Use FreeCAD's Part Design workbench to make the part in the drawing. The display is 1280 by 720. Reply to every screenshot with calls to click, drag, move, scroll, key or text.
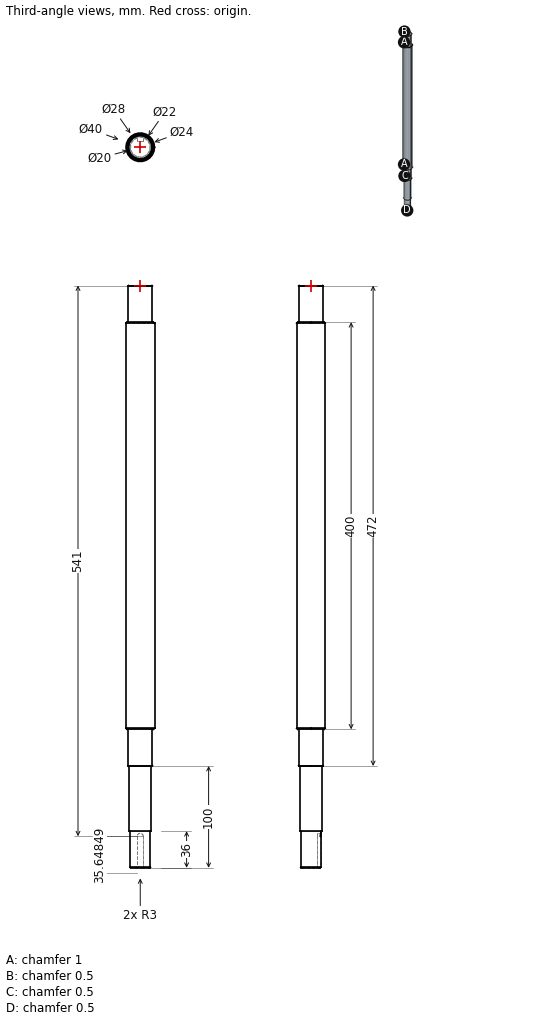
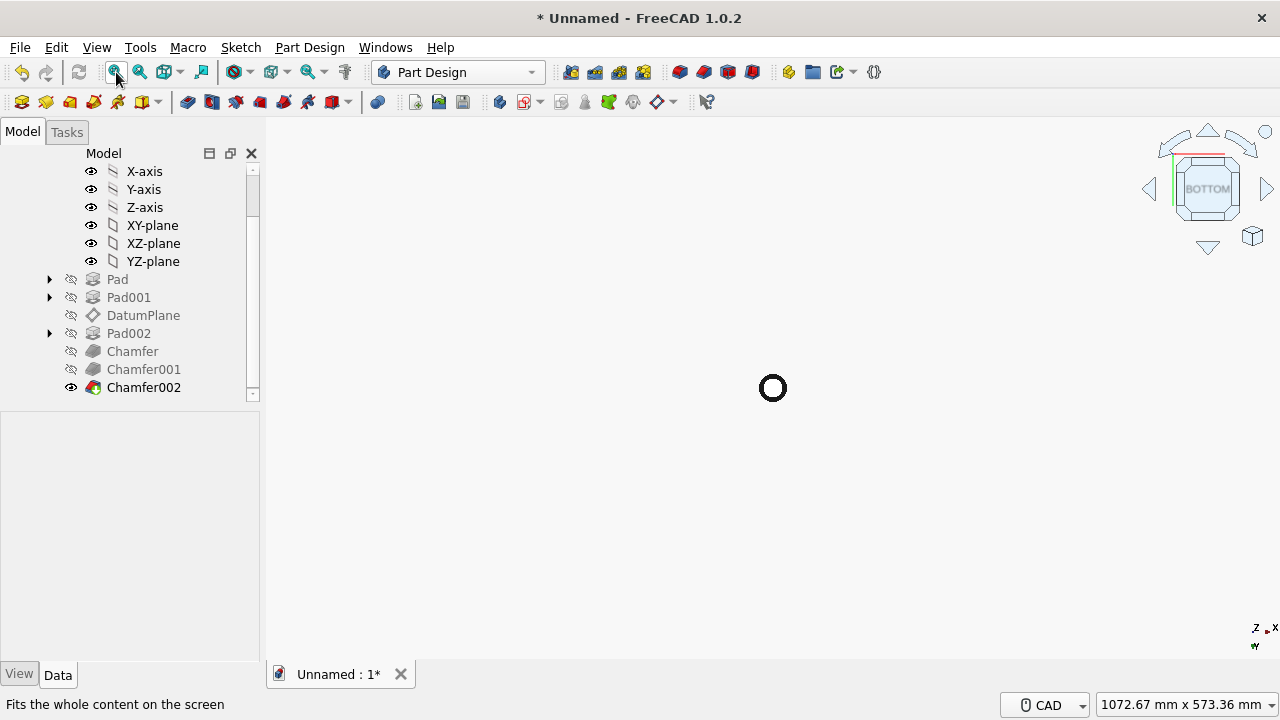
click(773, 387)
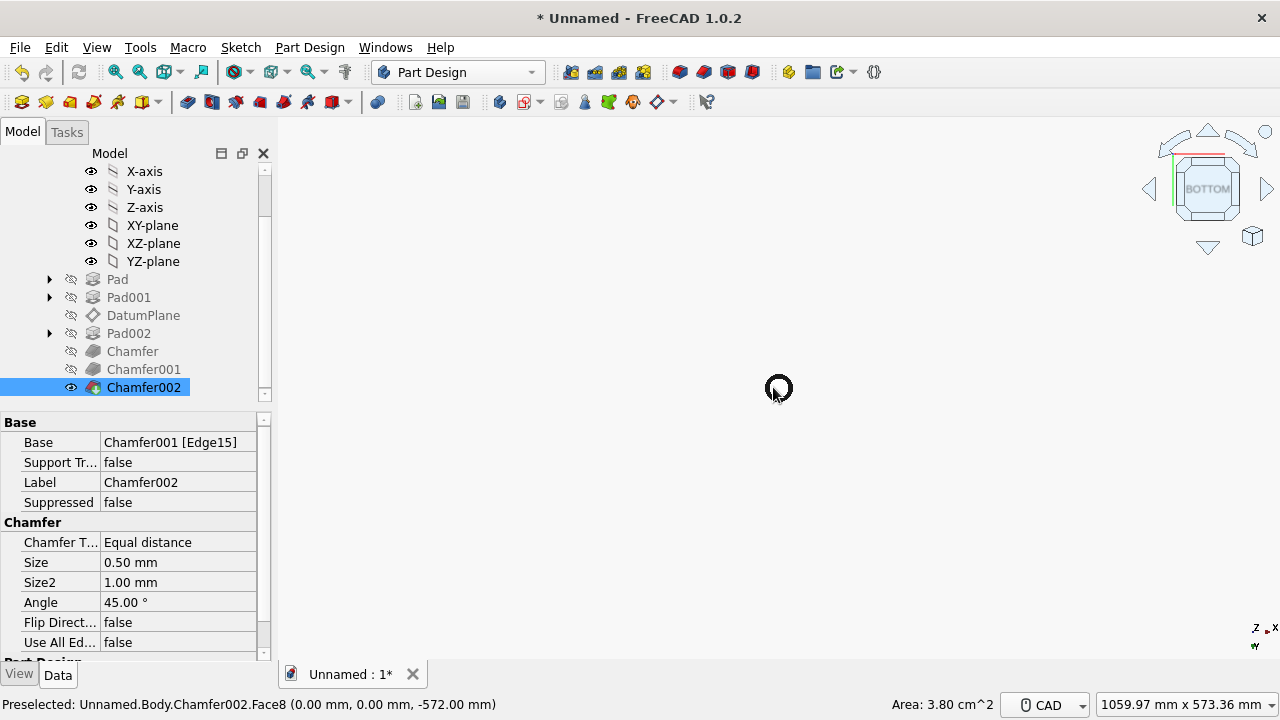
click(524, 102)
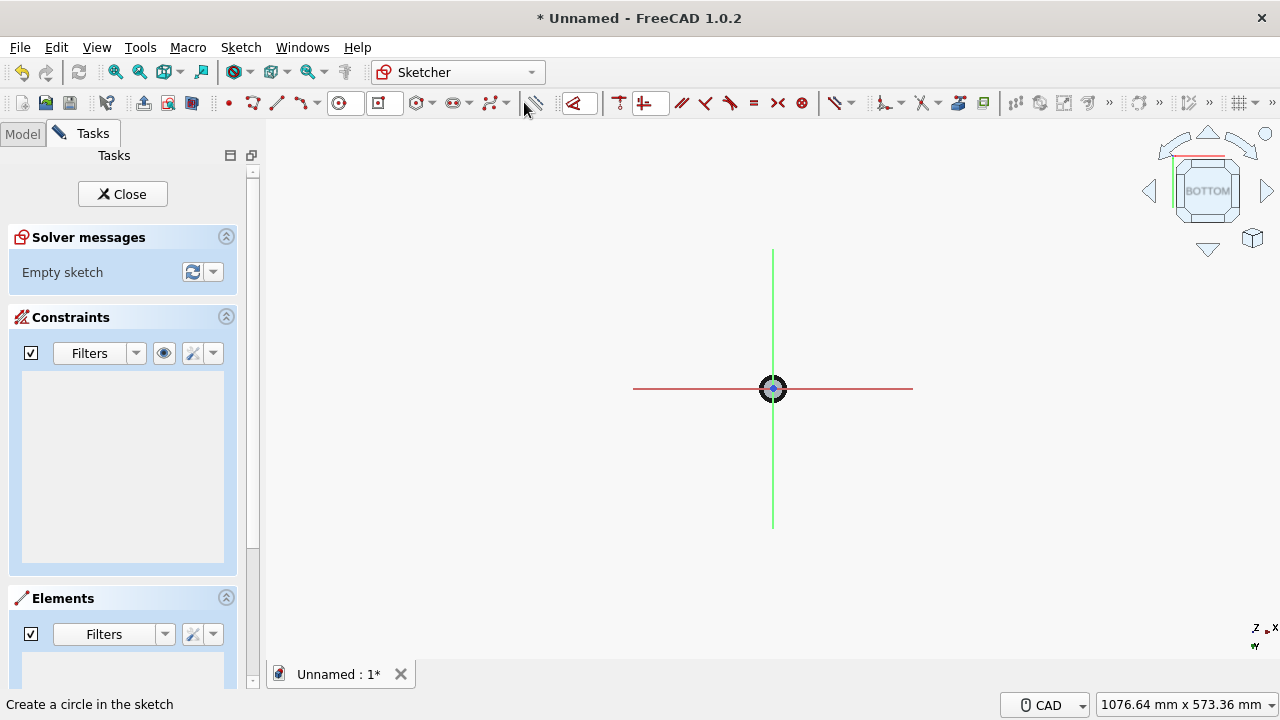
scroll(782, 389, up, 11)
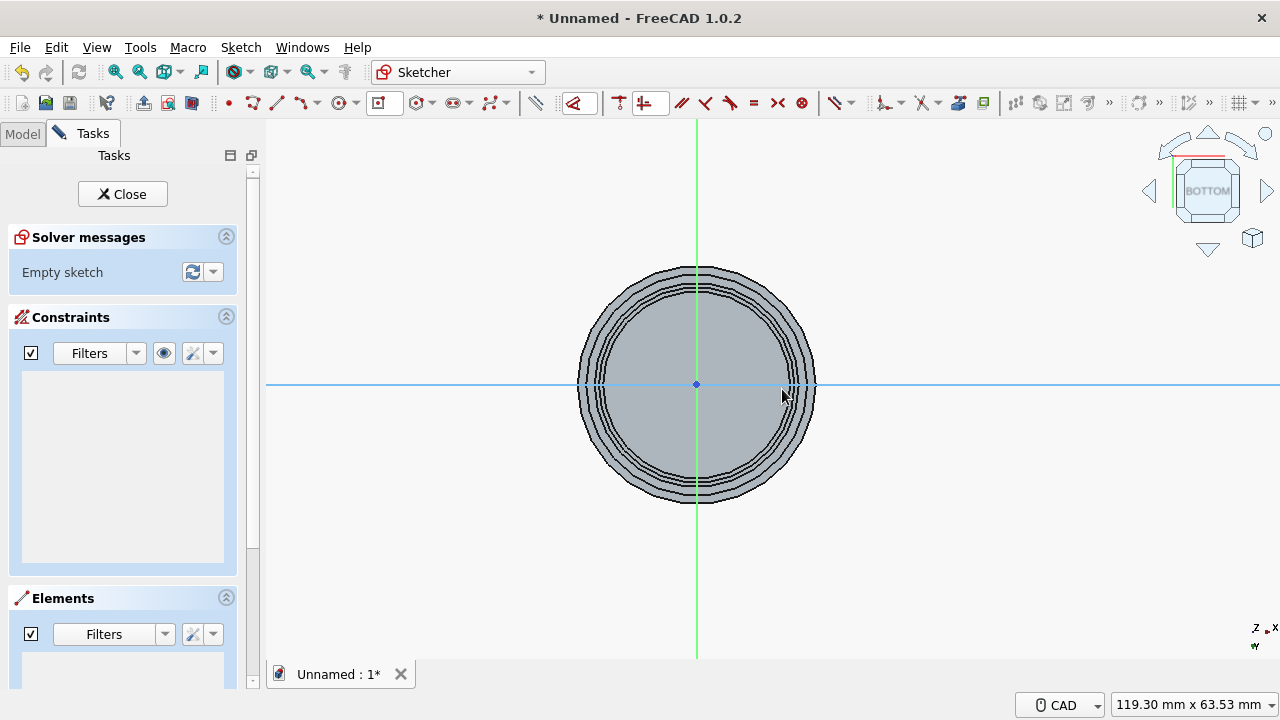
key(g)
key(c)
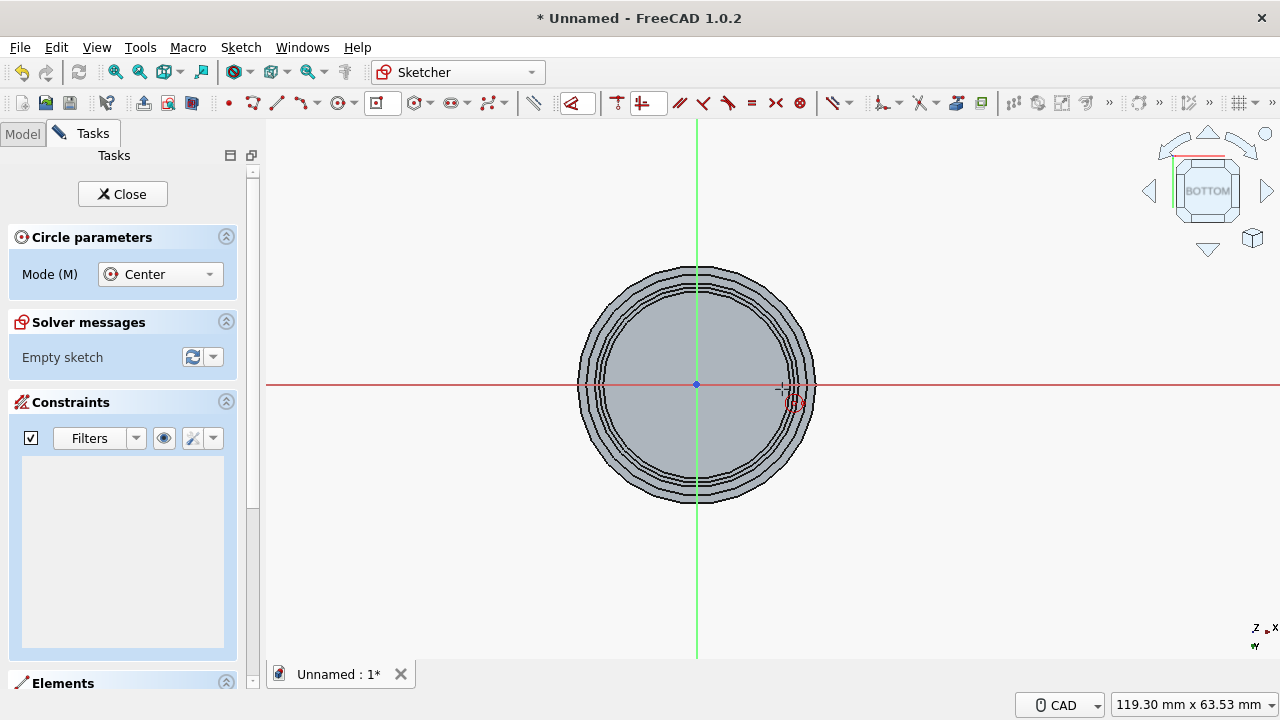
click(697, 385)
move(817, 265)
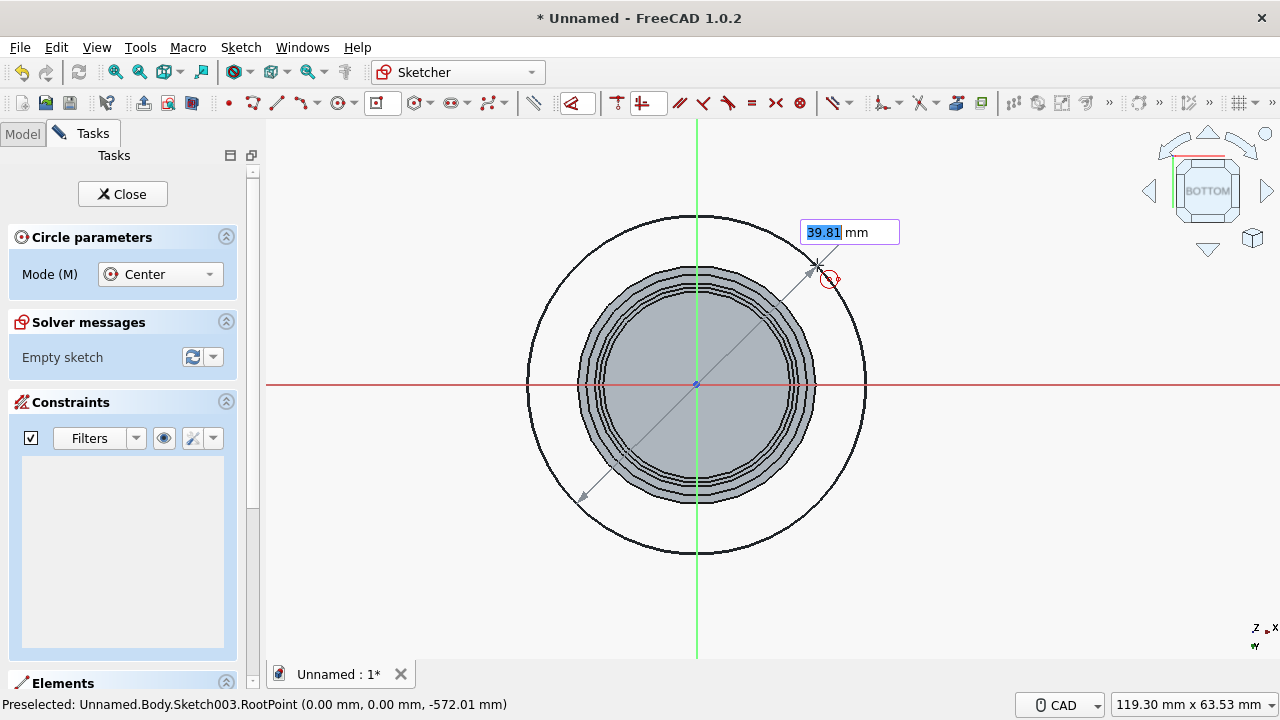
text(40)
key(Return)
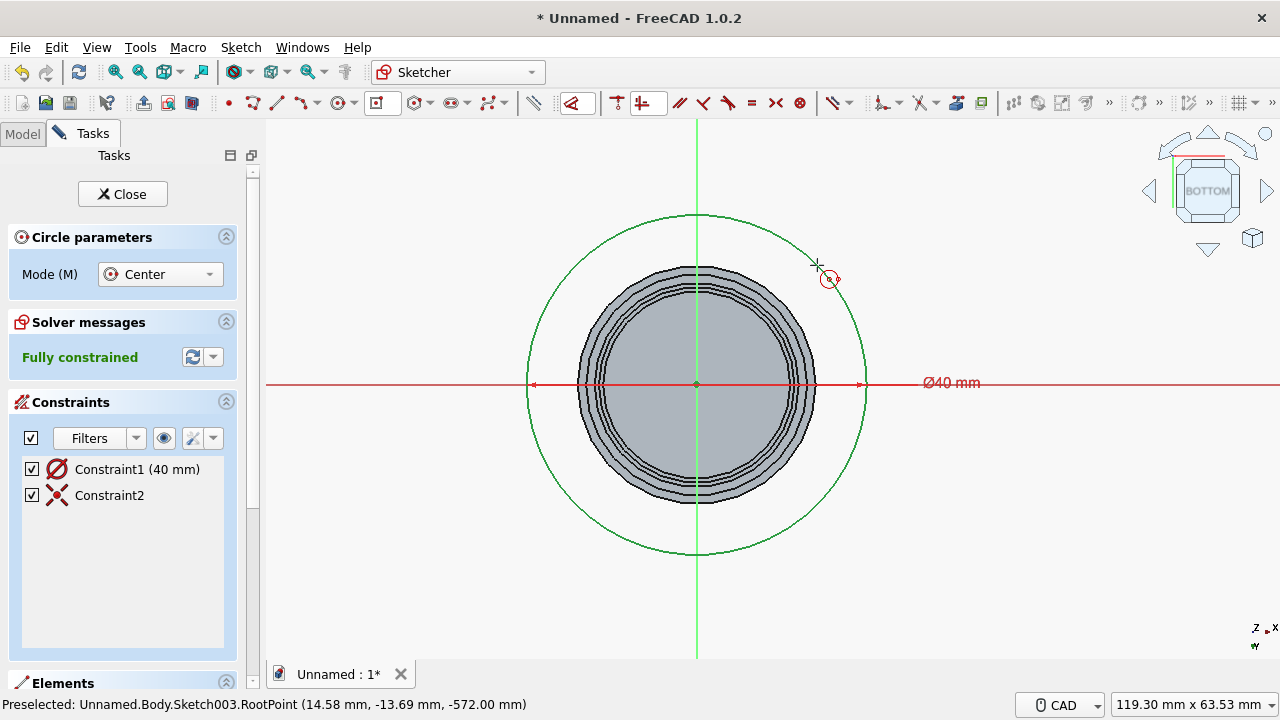
click(697, 385)
move(757, 325)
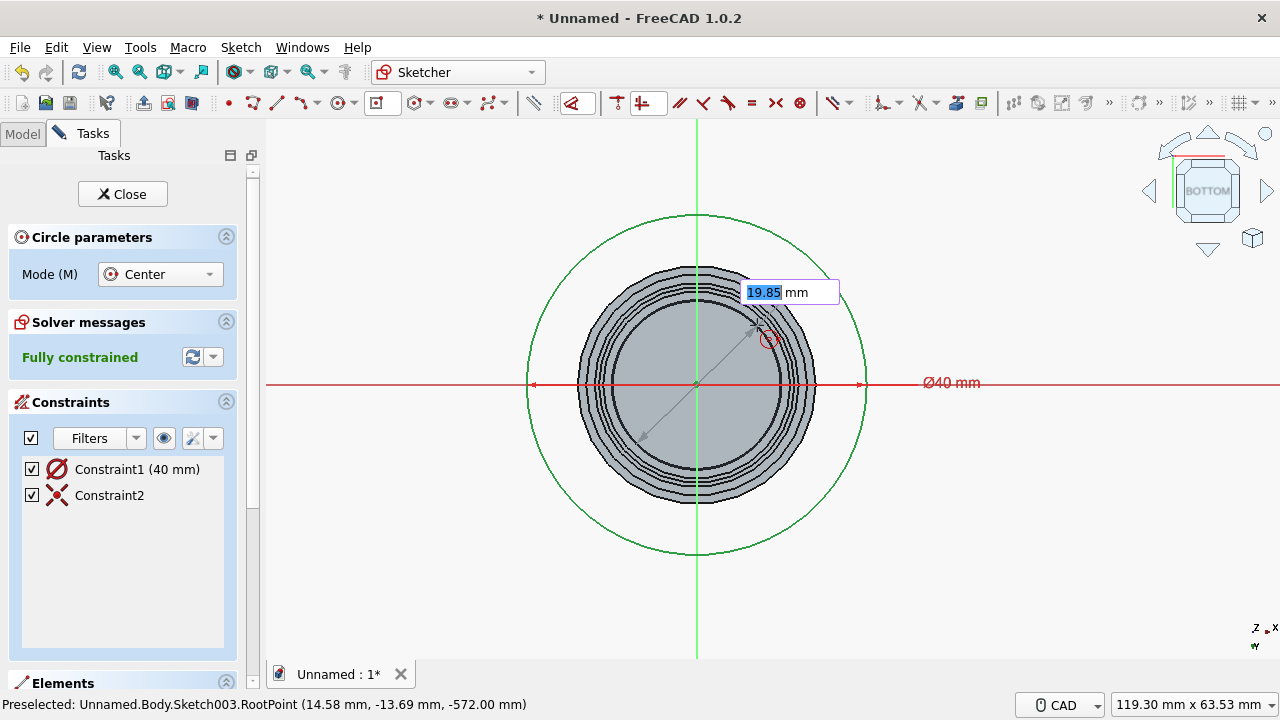
text(20)
key(Return)
key(Escape)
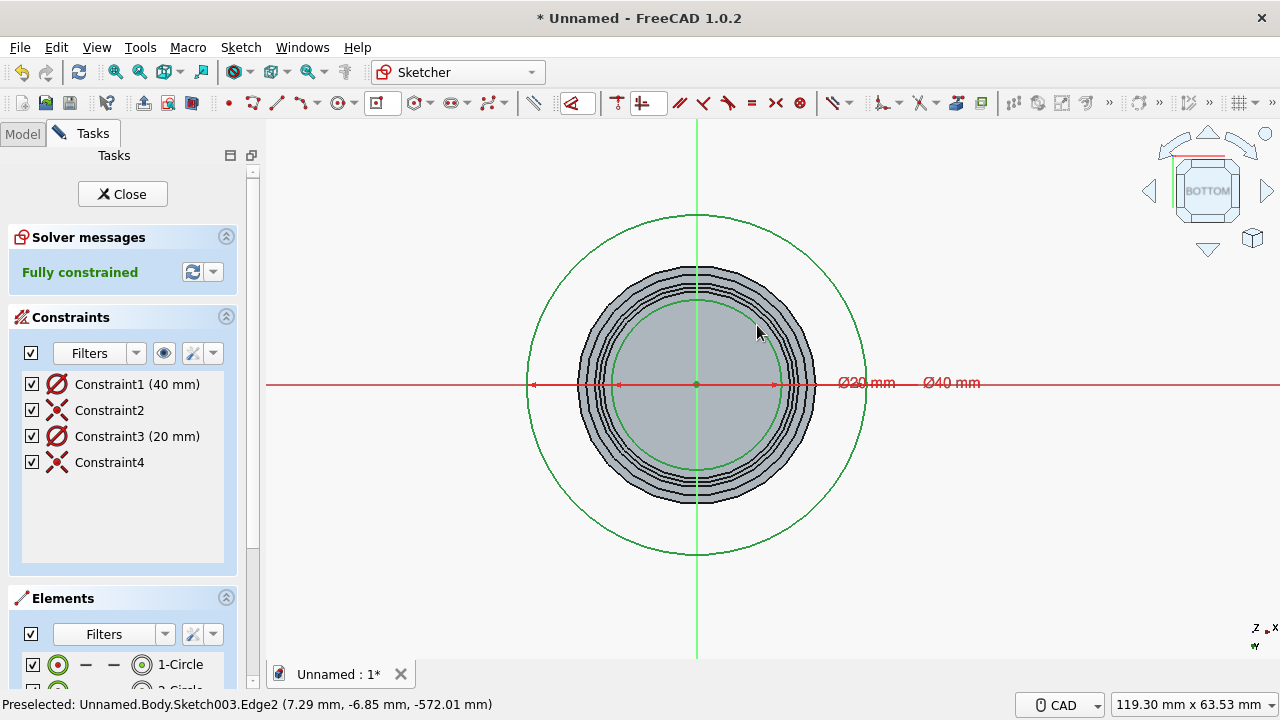
click(123, 194)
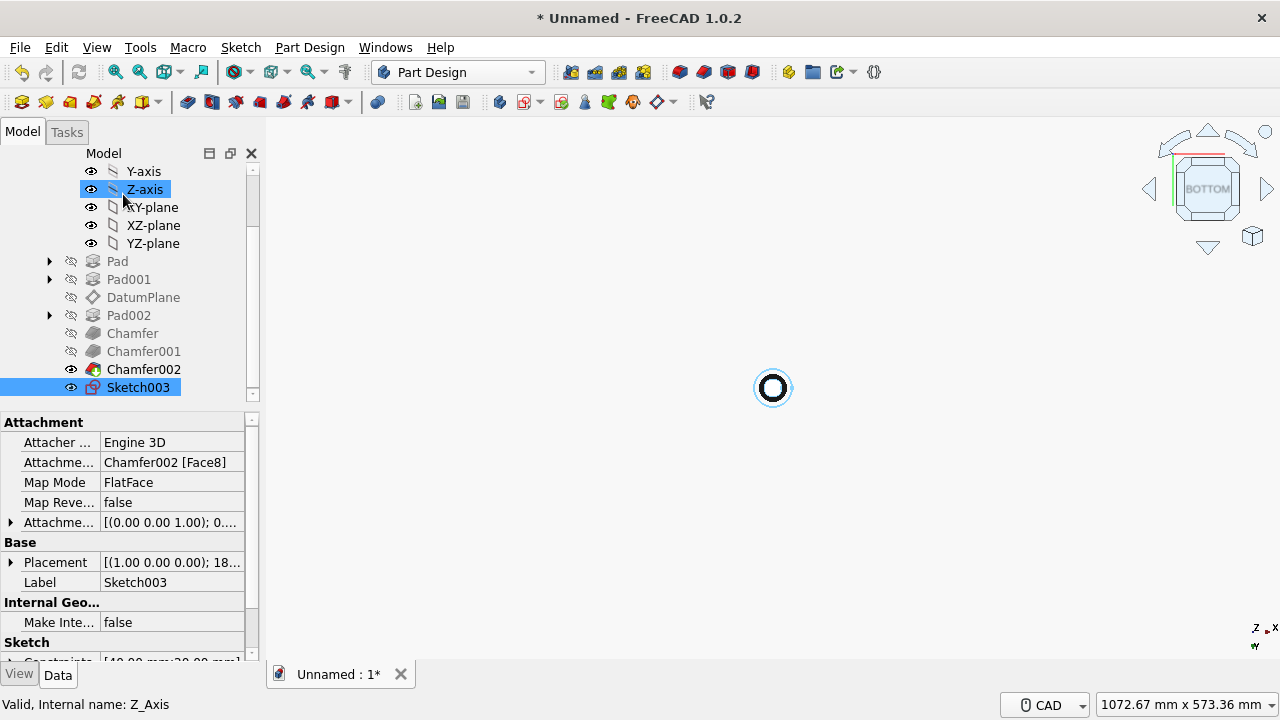
click(188, 102)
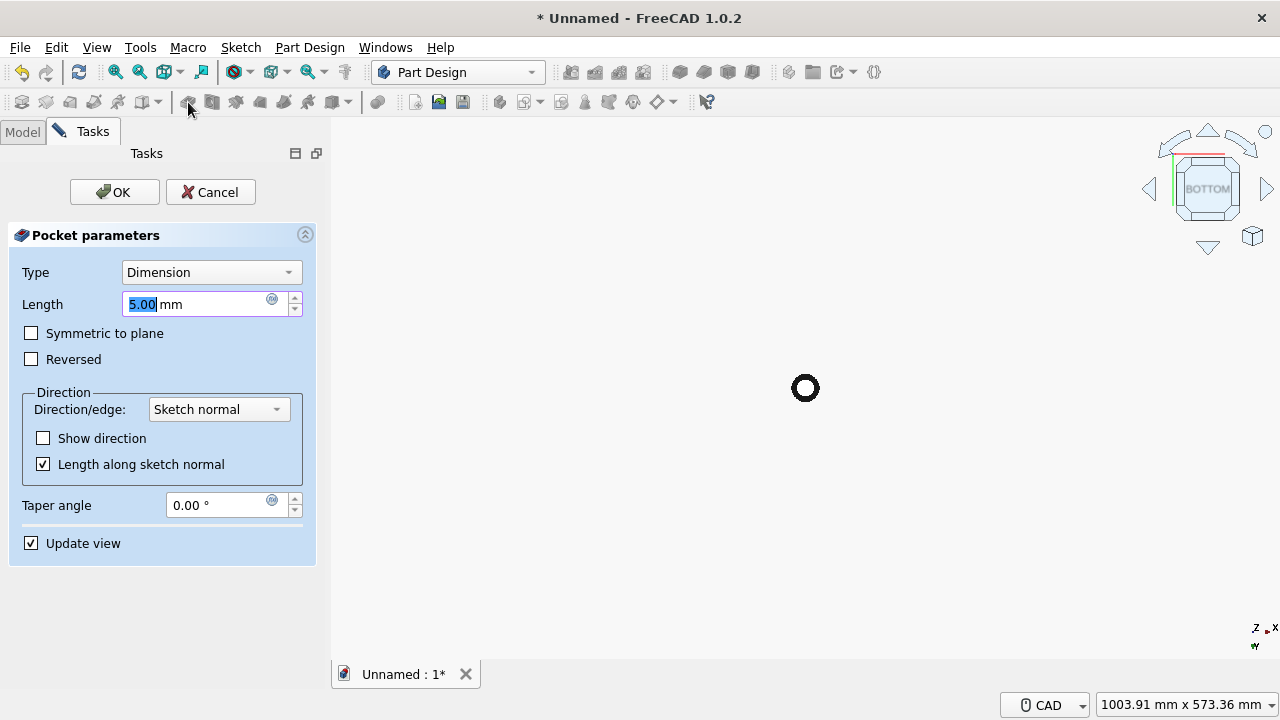
text(36)
key(Tab)